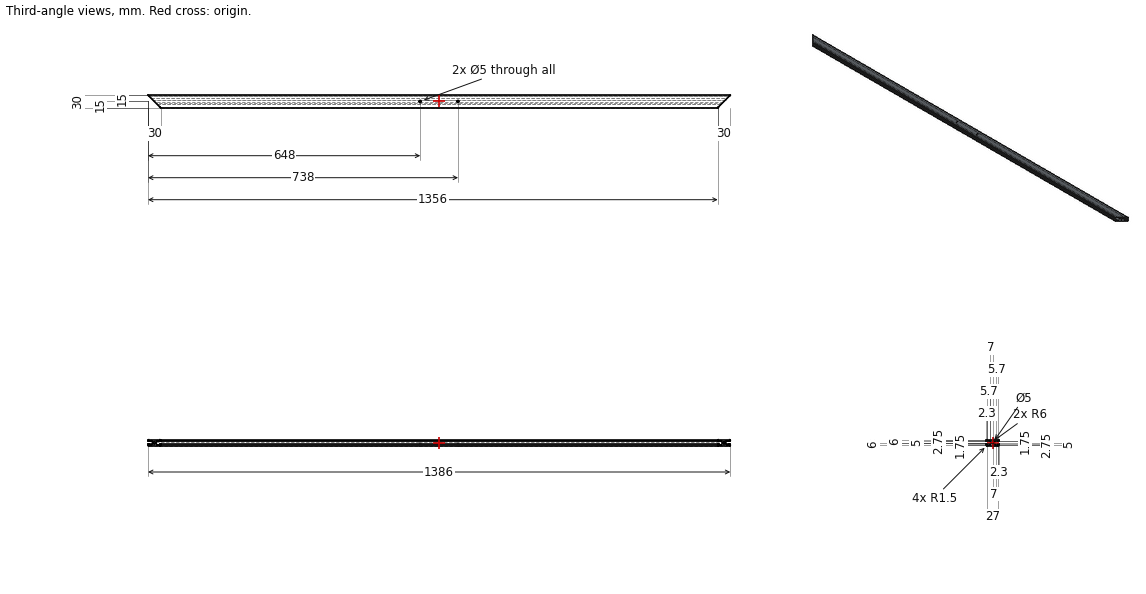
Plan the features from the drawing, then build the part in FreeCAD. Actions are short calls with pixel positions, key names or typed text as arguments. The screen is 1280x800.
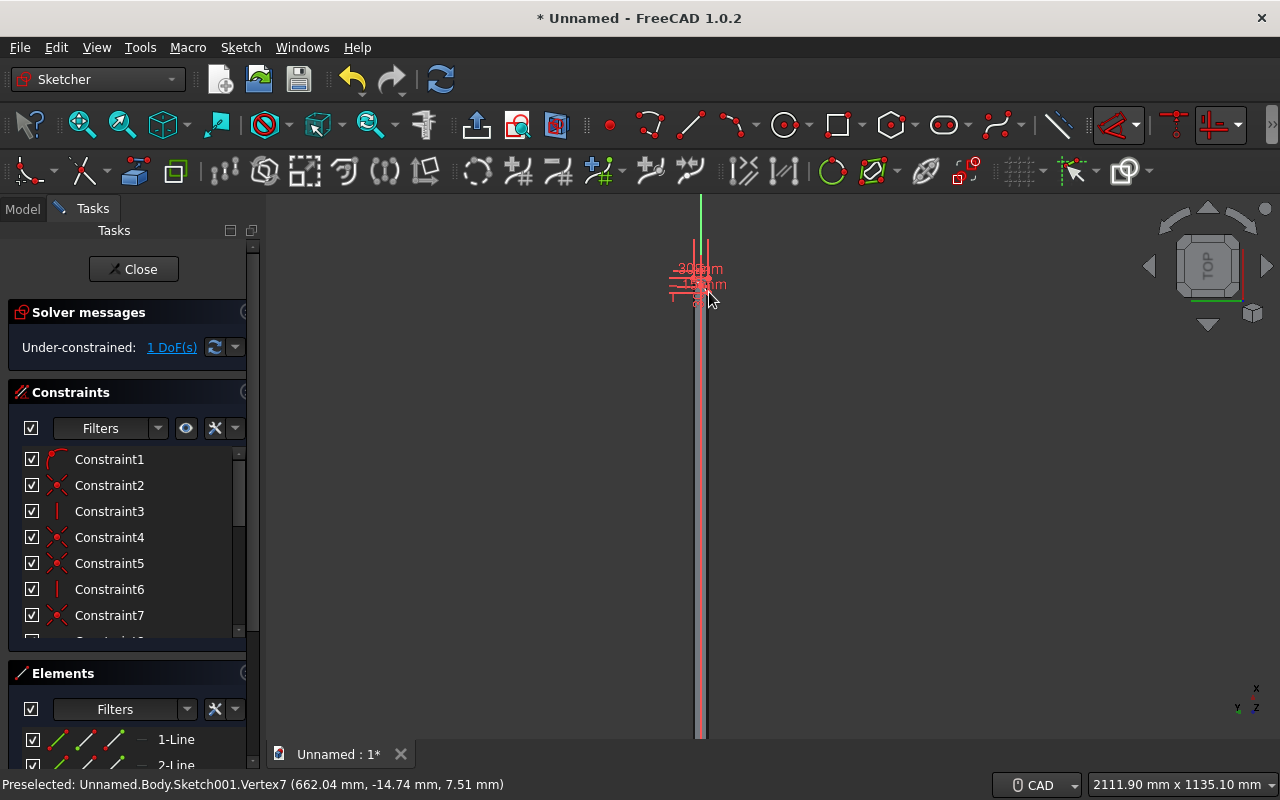
click(708, 293)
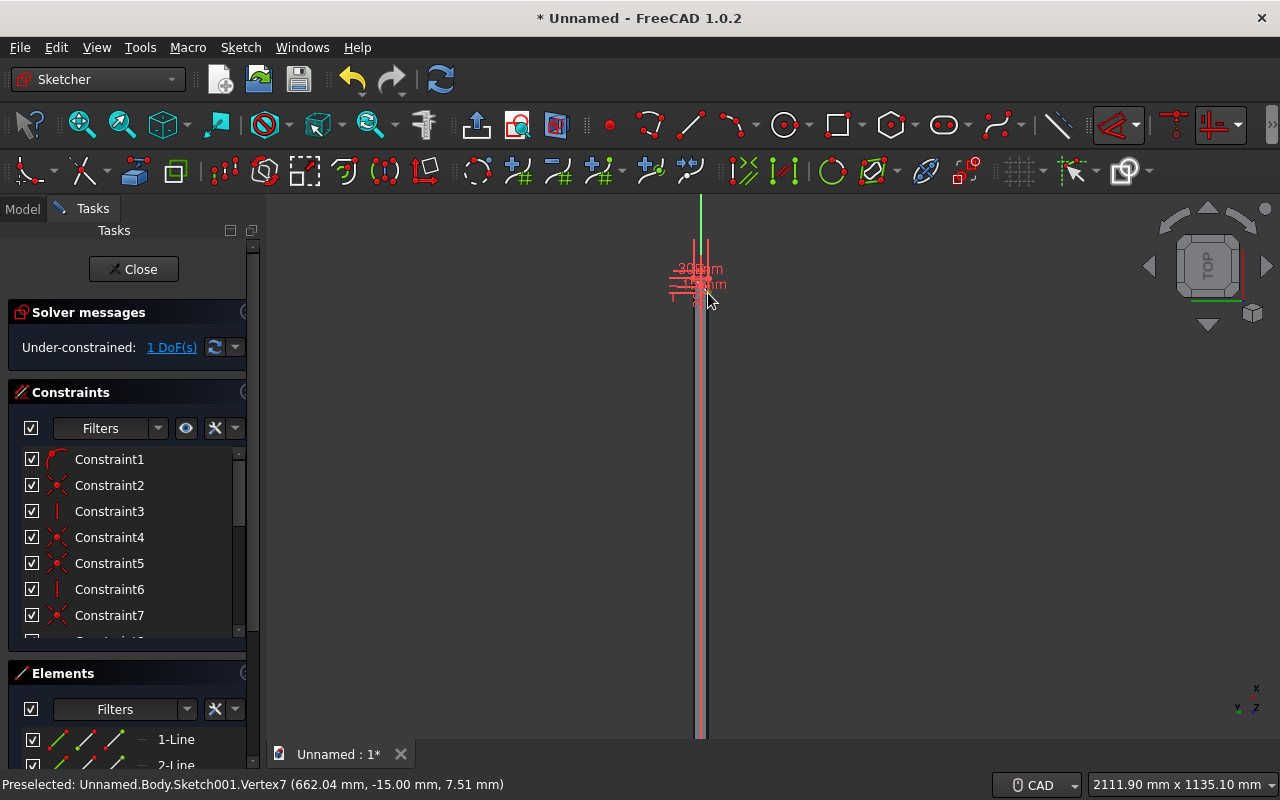
click(1138, 126)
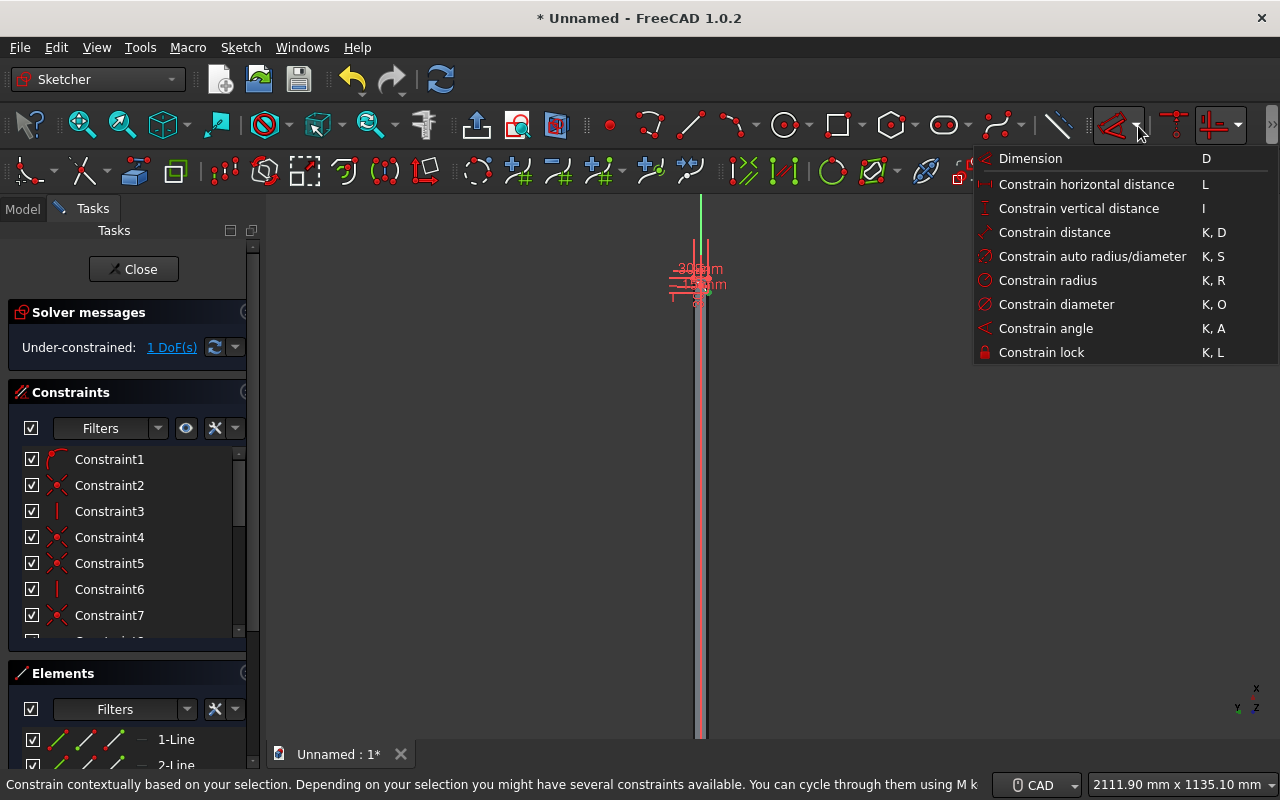
click(1126, 208)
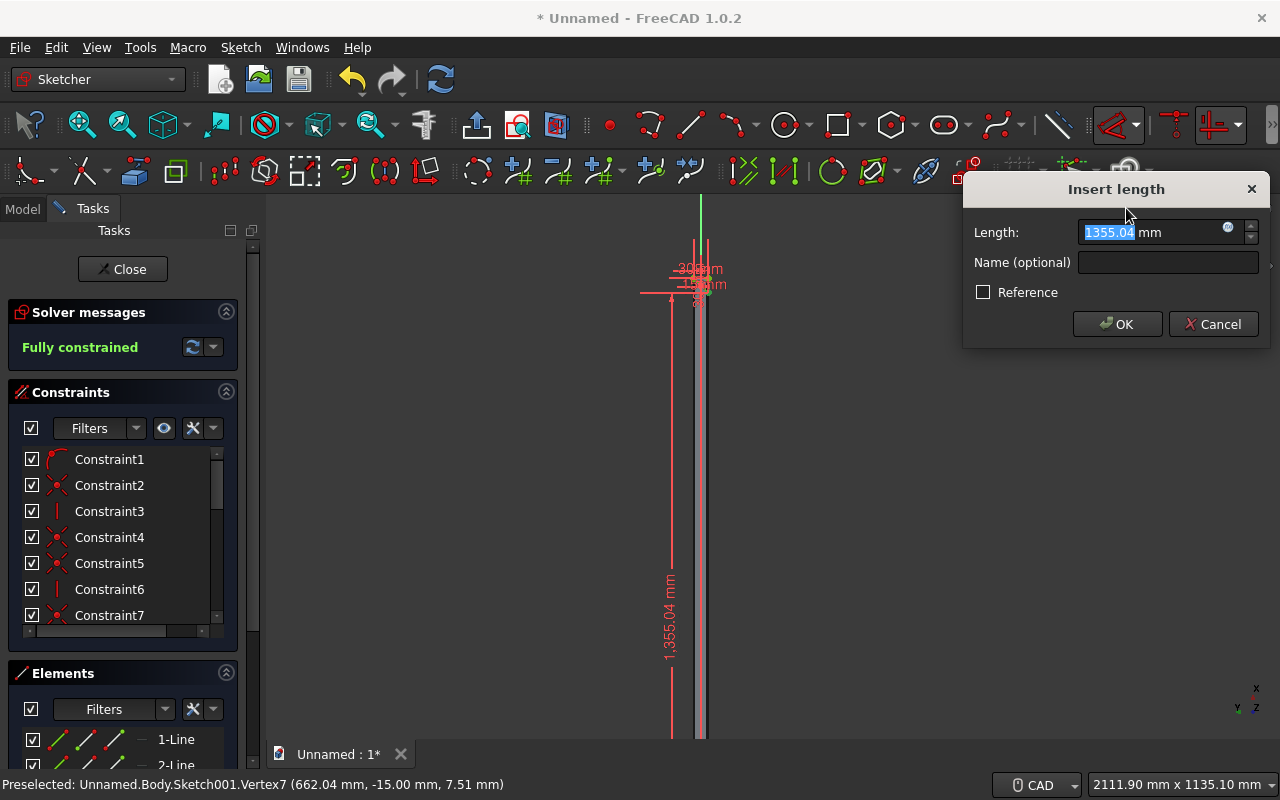
text(1356)
key(Return)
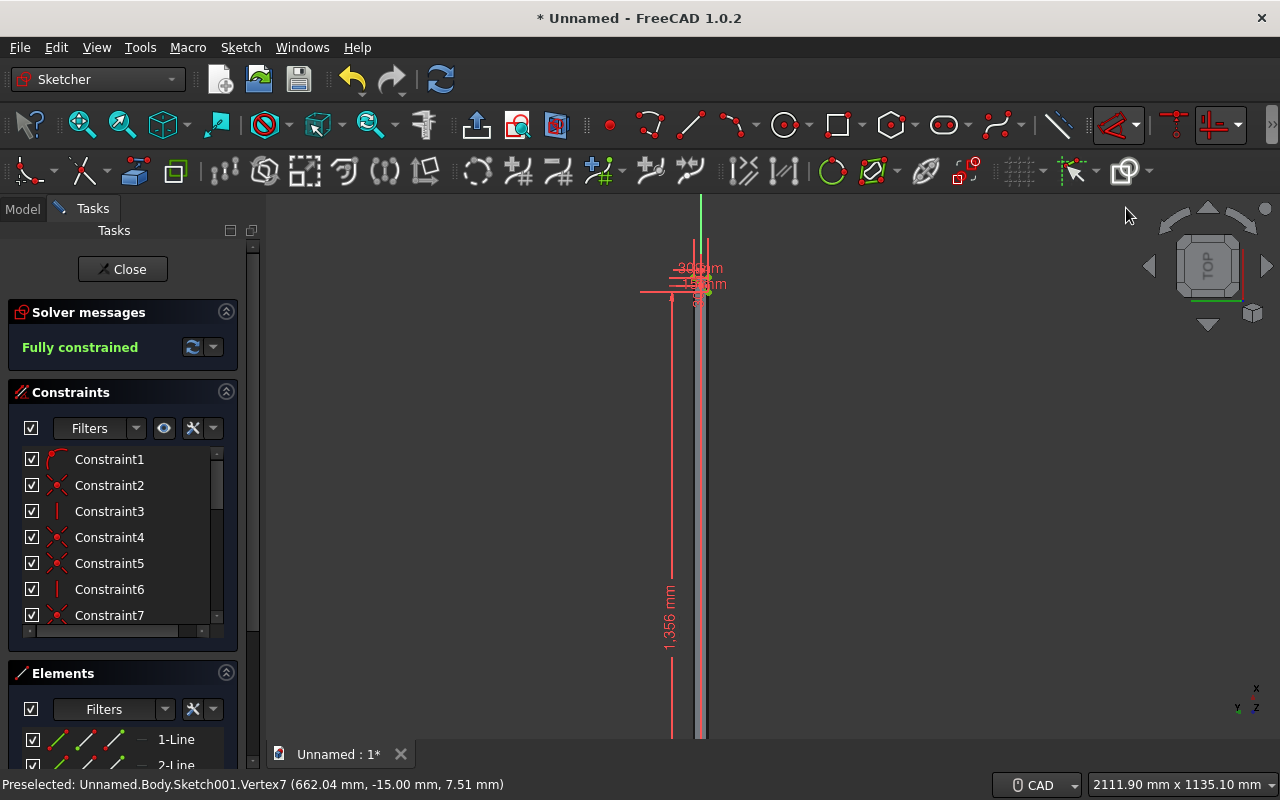
click(123, 269)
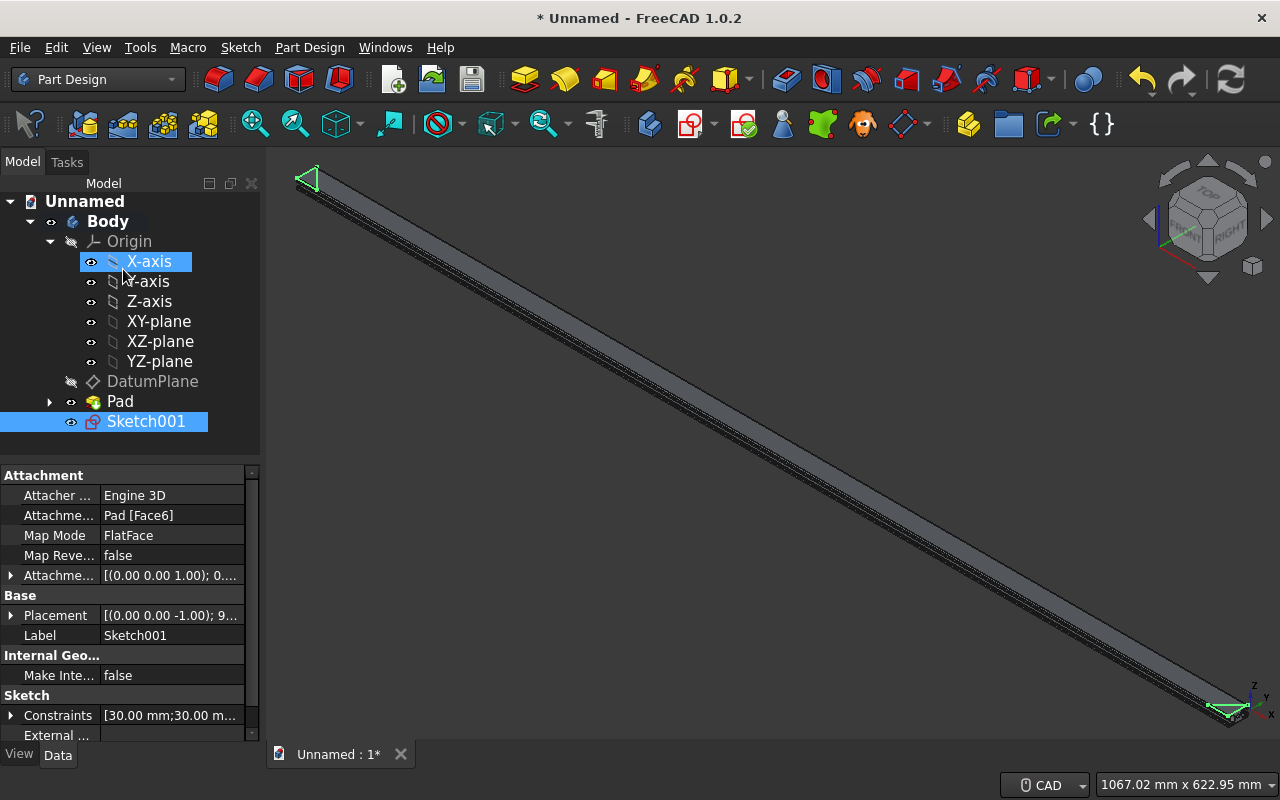
click(788, 80)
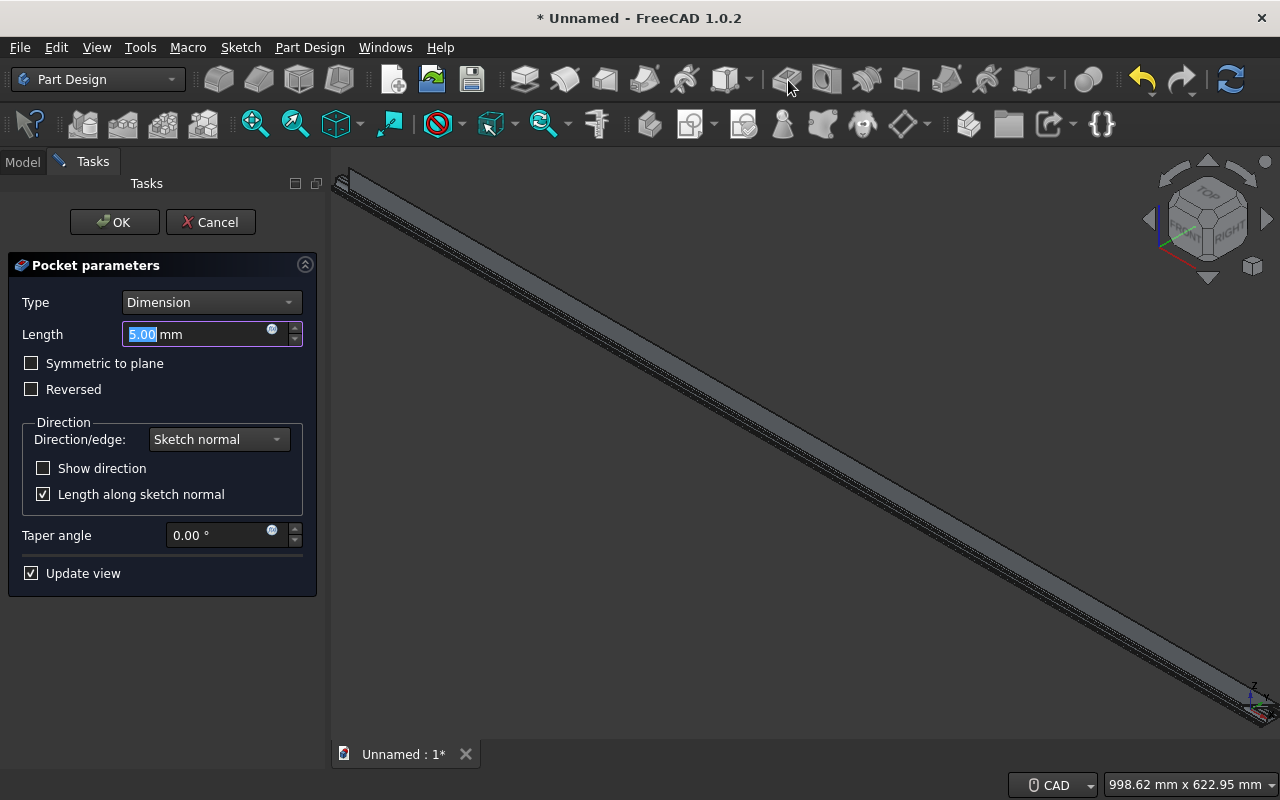
click(212, 302)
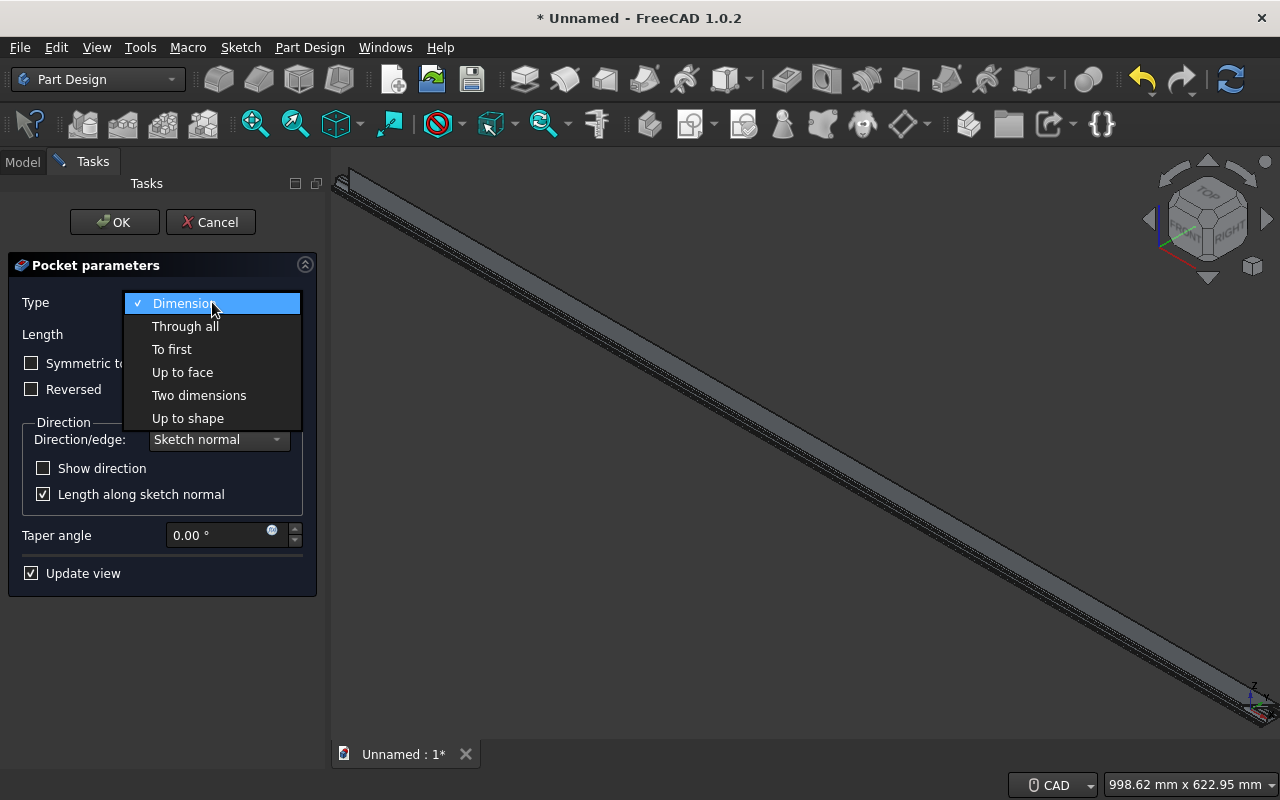
click(212, 326)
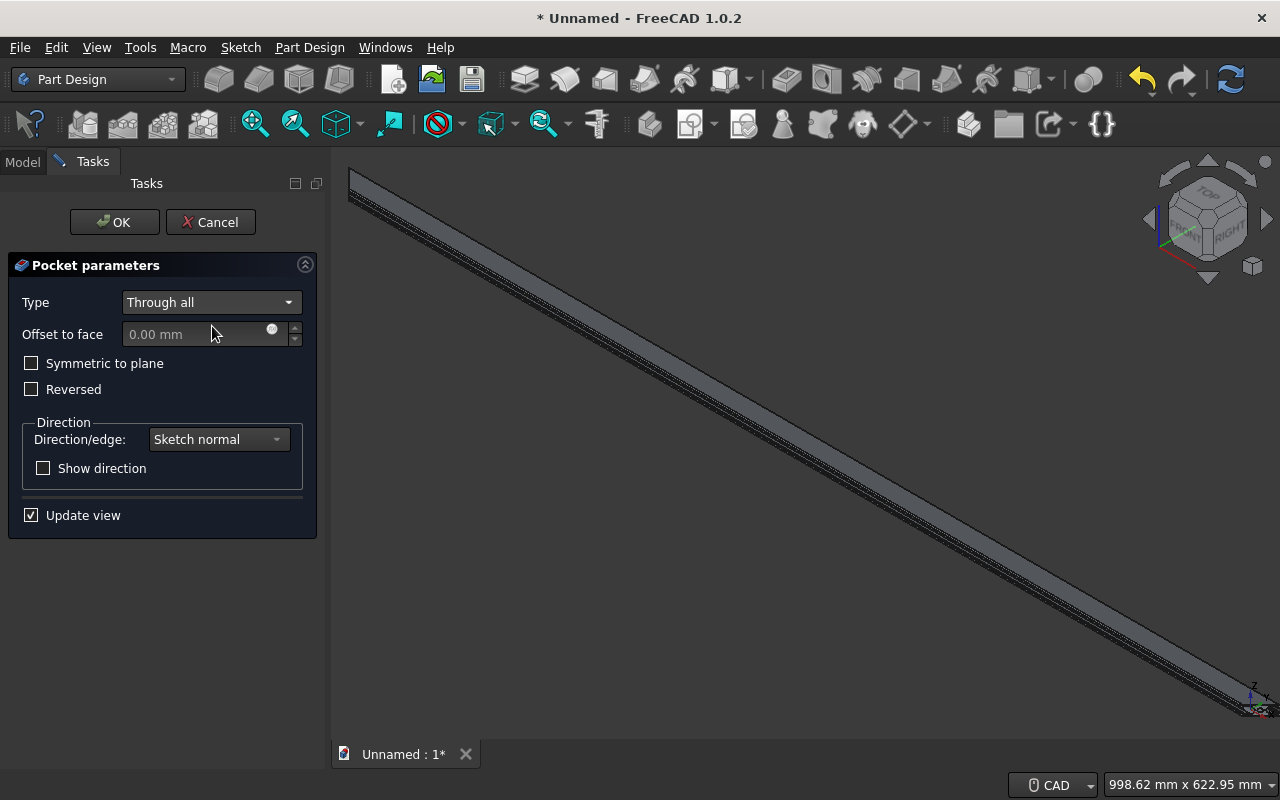
click(115, 222)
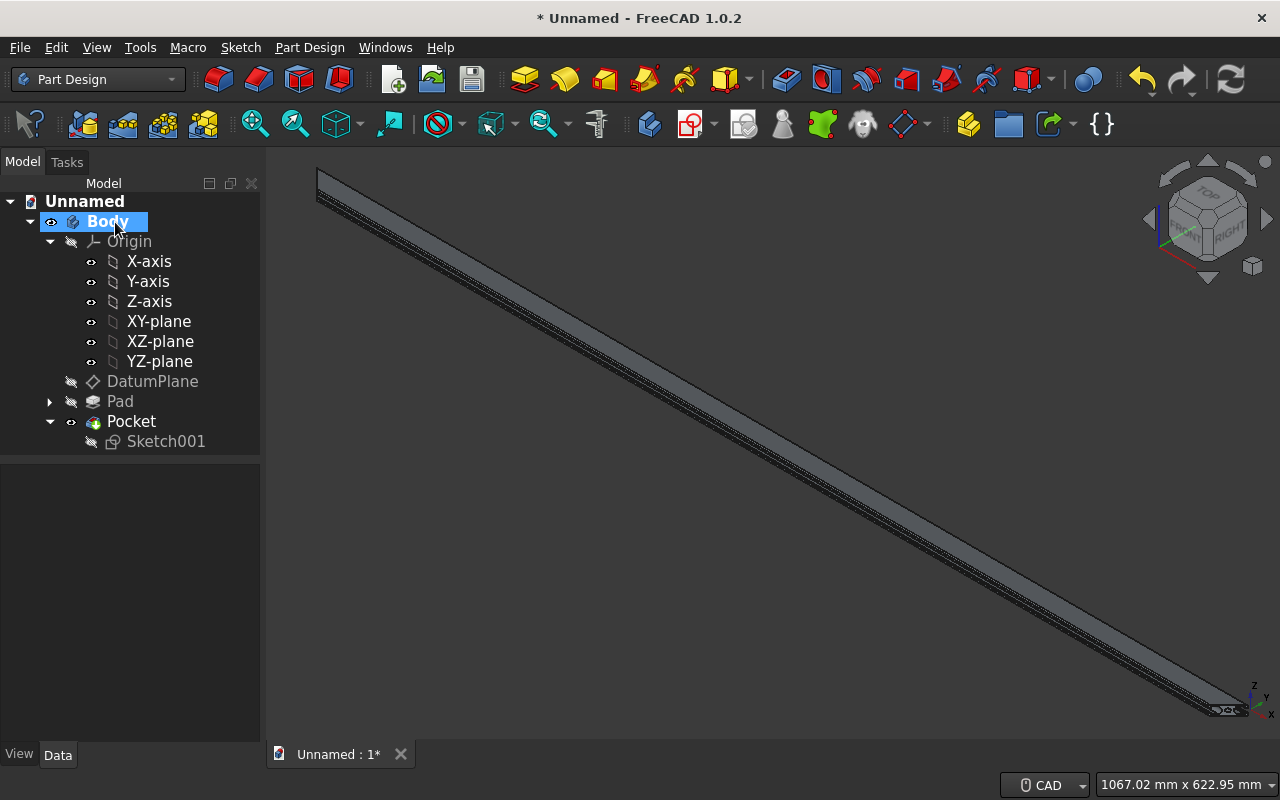
click(905, 517)